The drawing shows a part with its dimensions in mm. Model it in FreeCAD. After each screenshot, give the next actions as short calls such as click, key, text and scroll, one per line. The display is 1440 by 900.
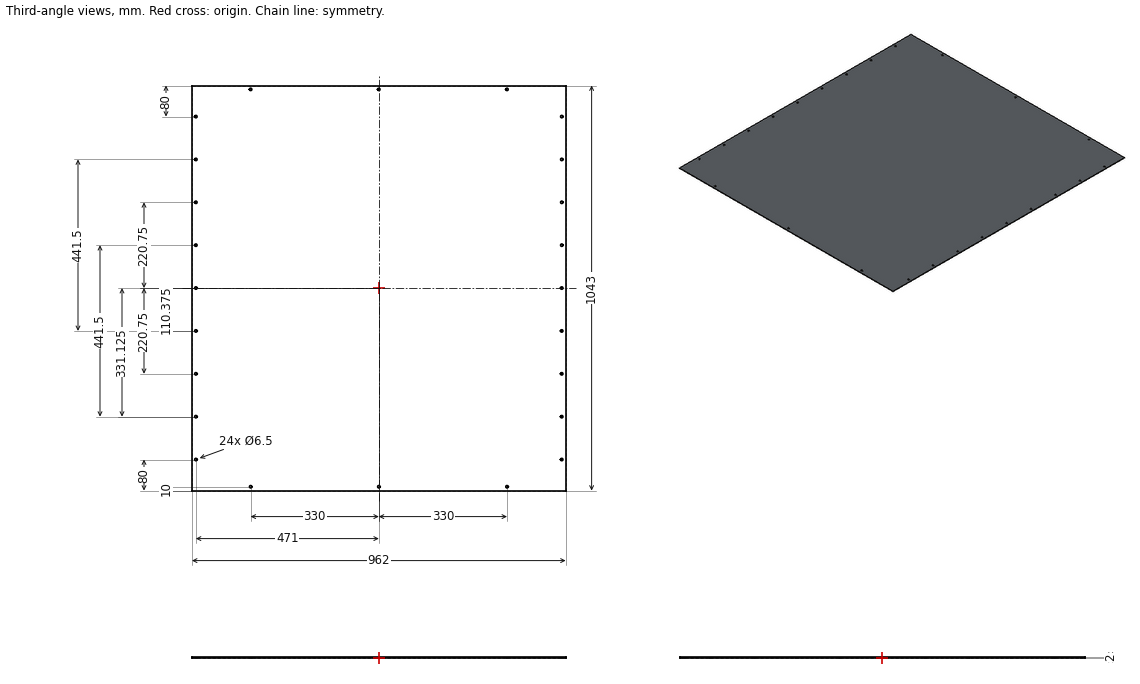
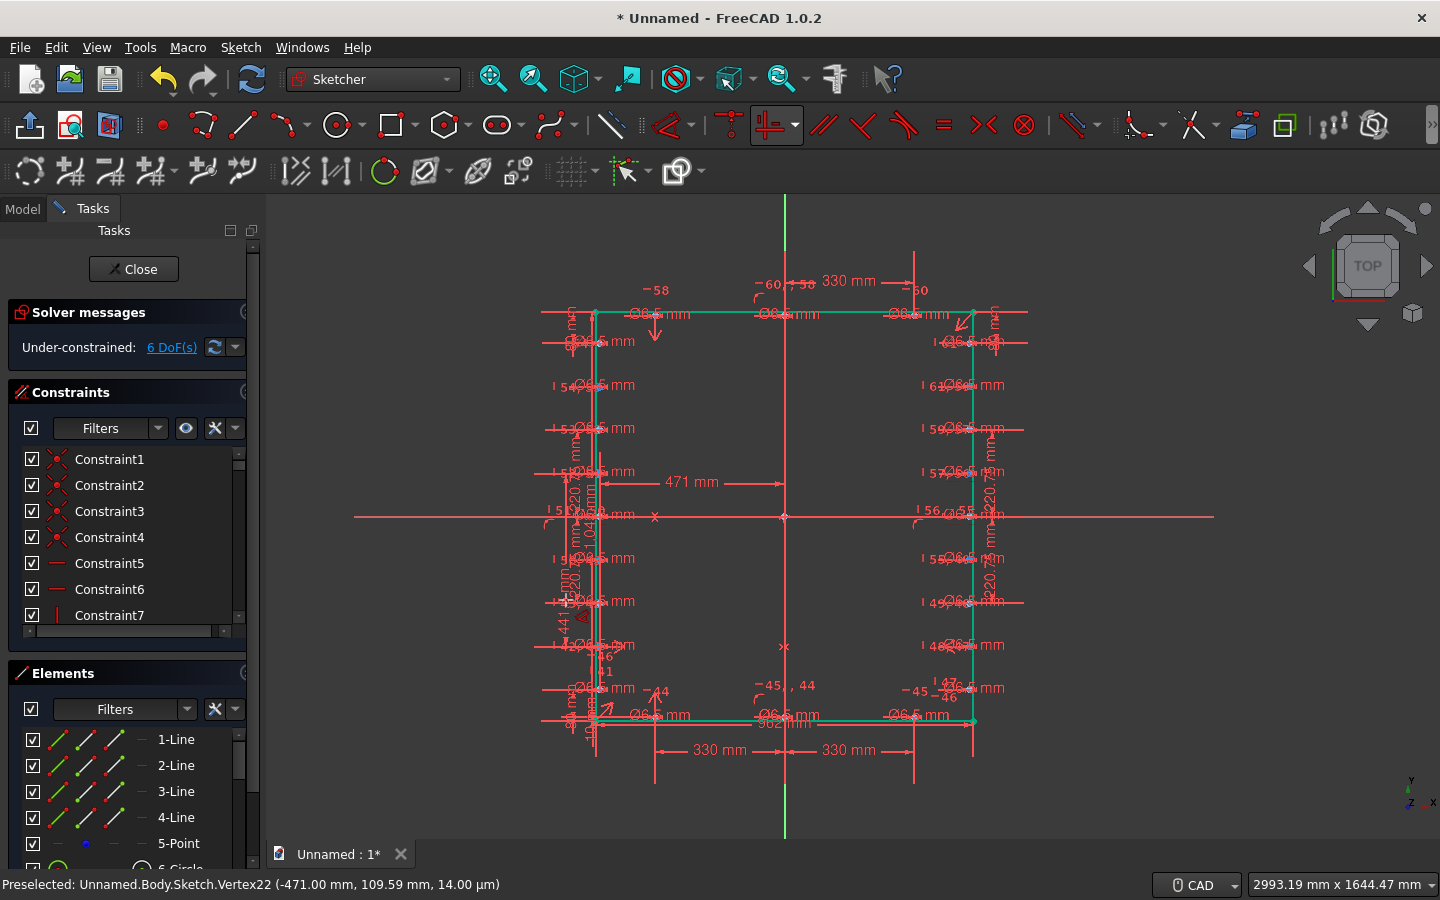
click(600, 560)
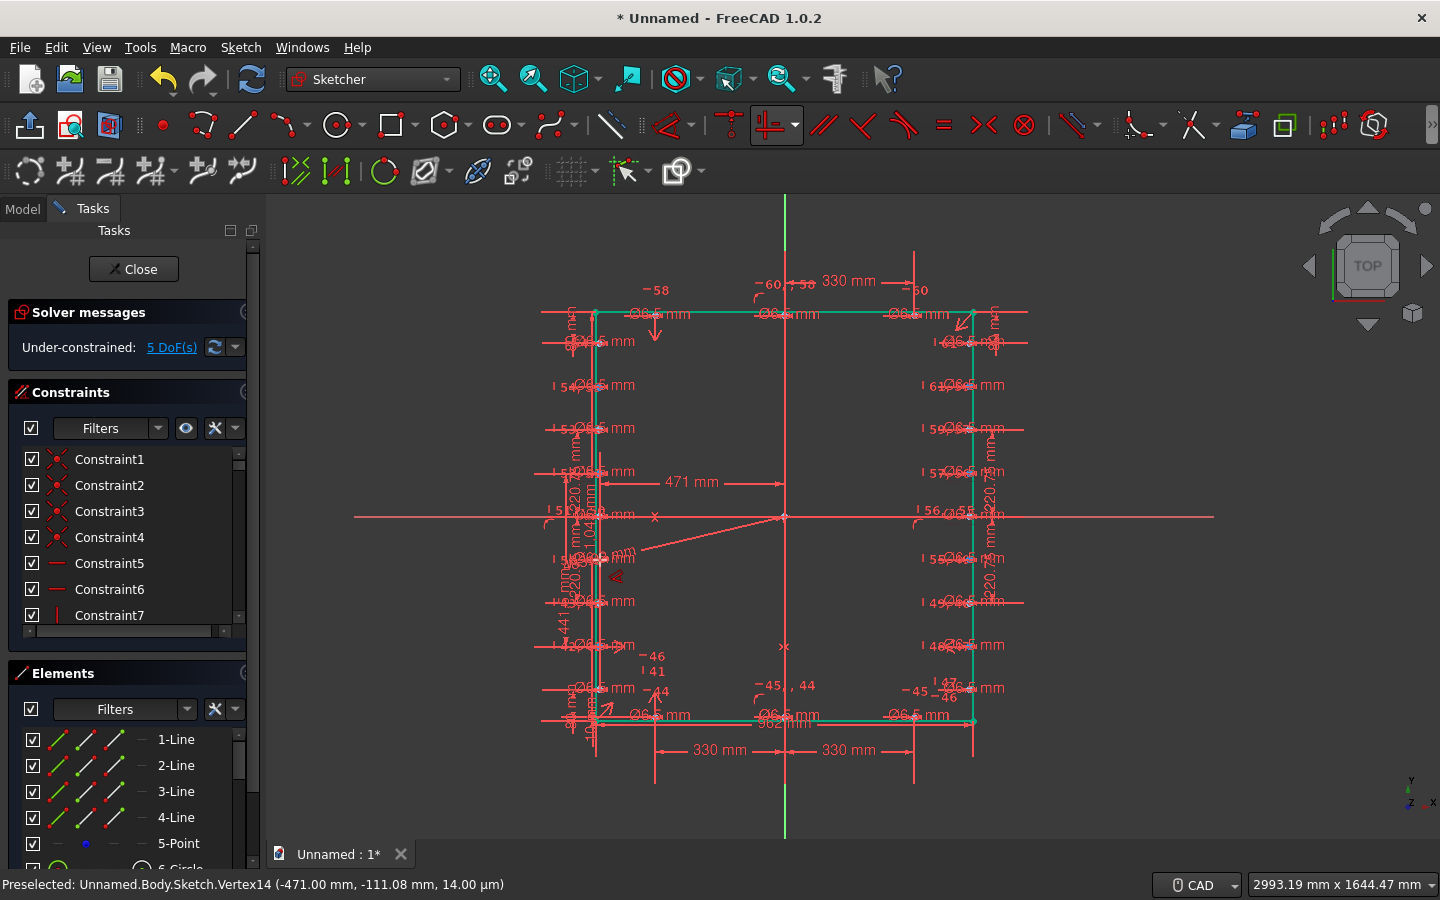
click(600, 387)
click(566, 434)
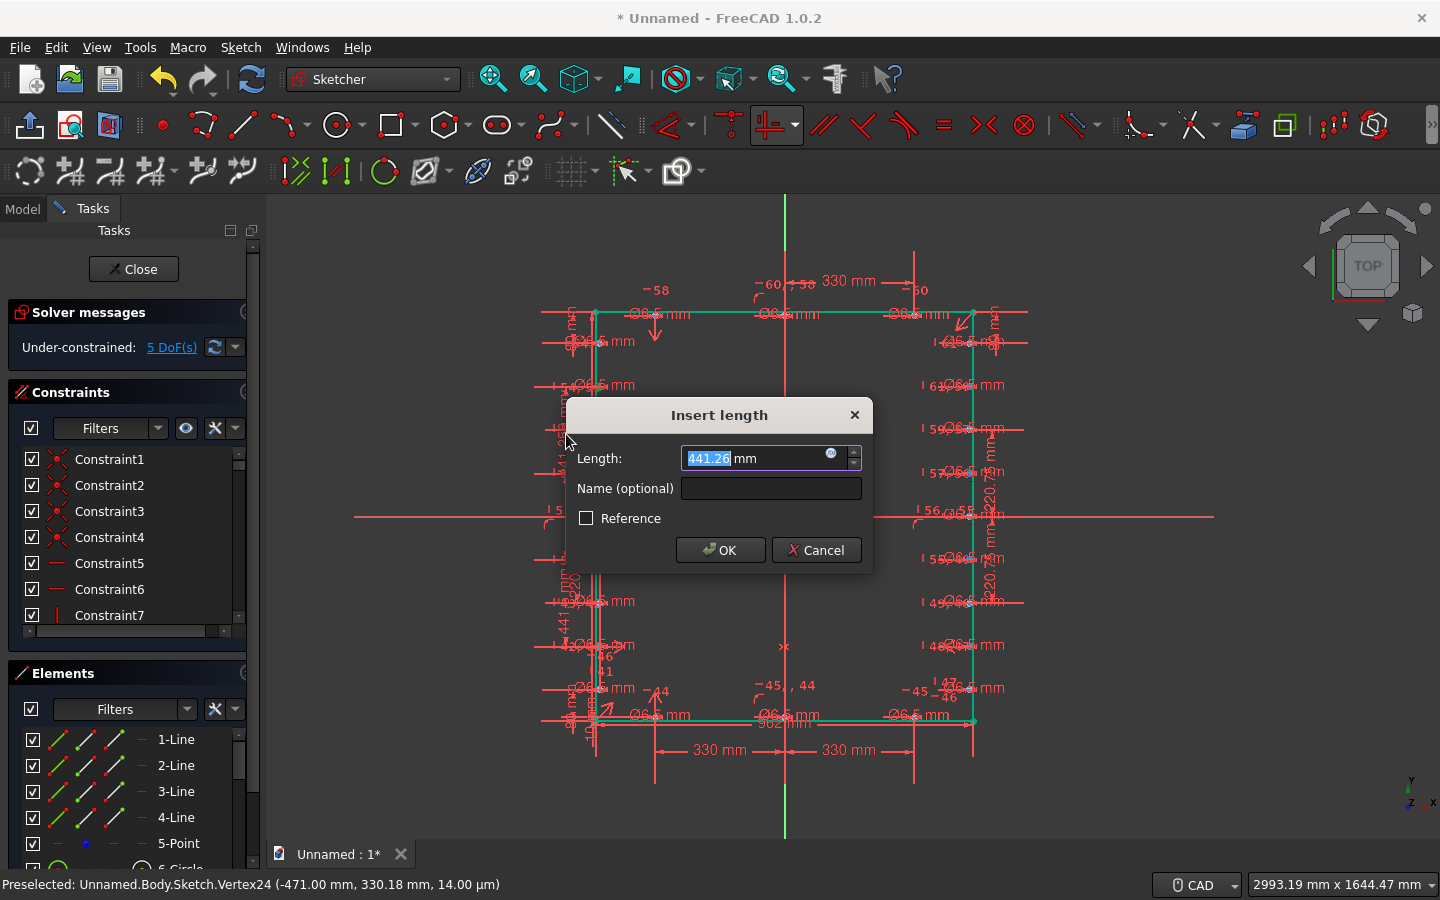
text(441.5)
key(Return)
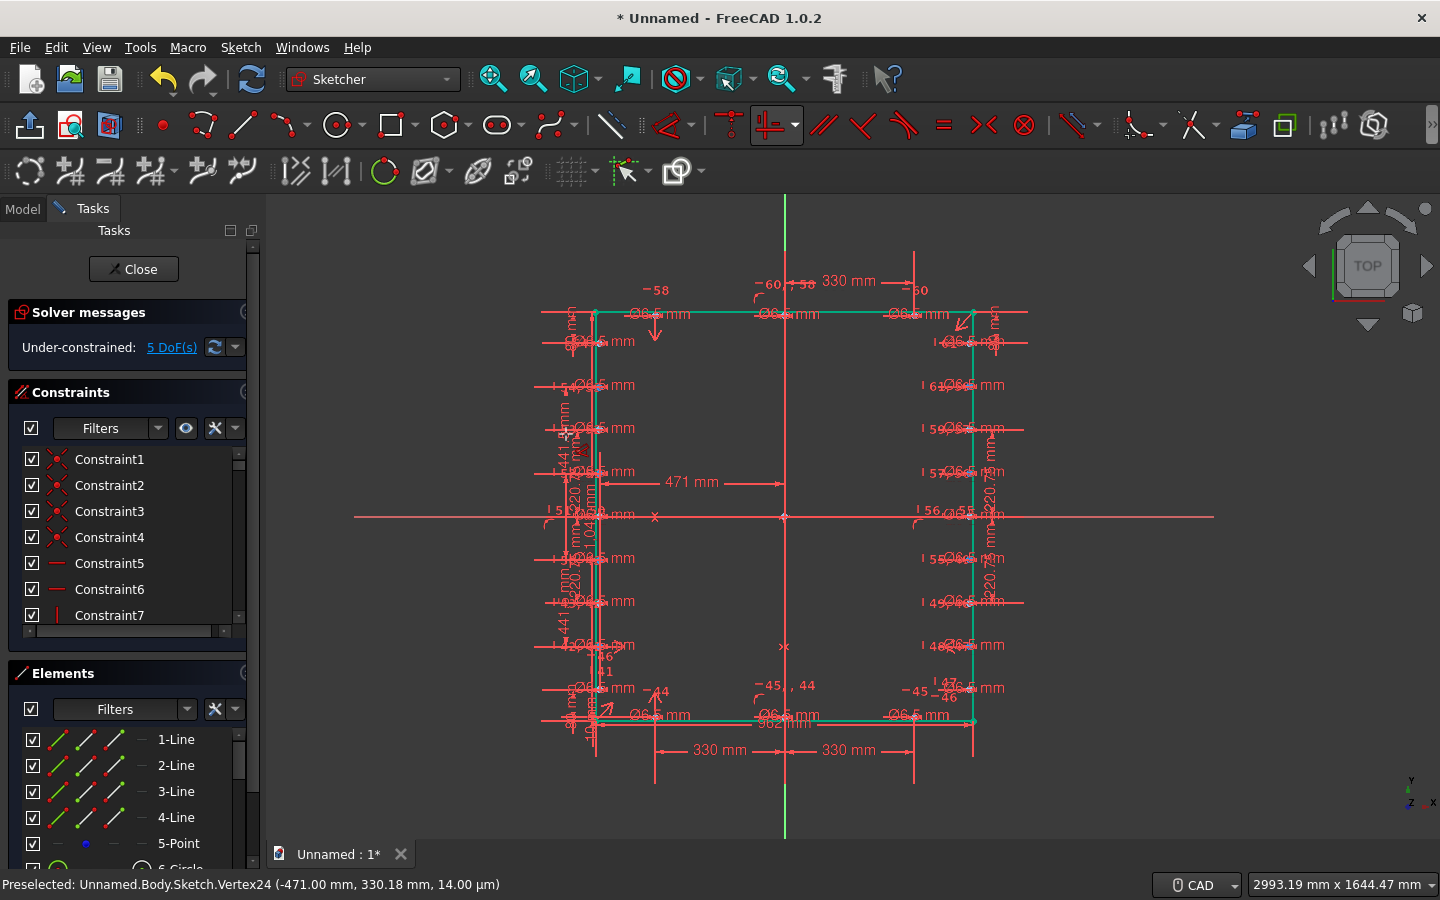
click(969, 647)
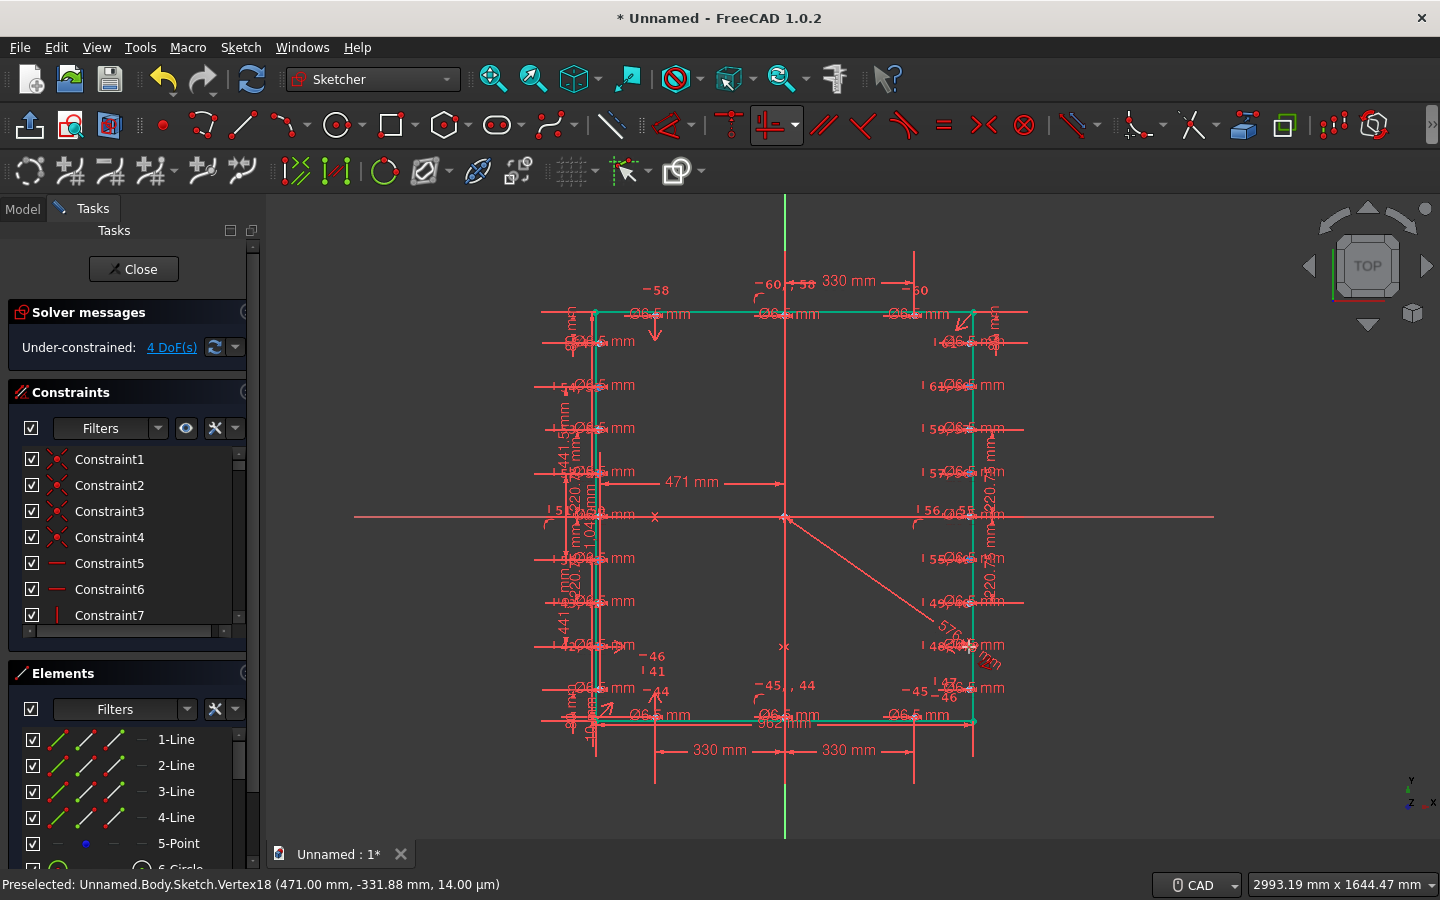
click(969, 474)
click(1003, 600)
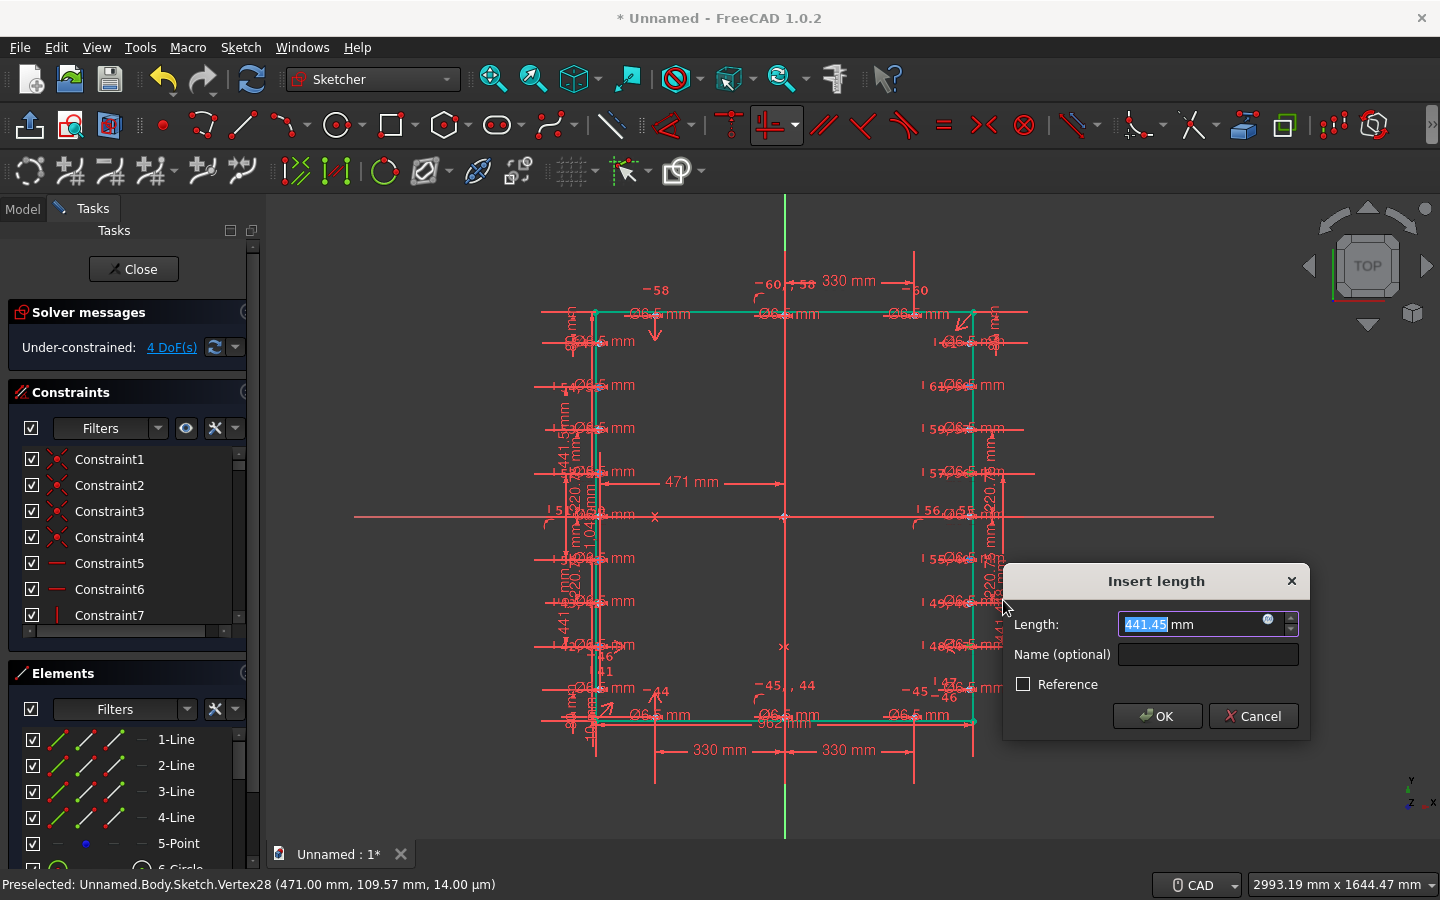
text(441.5)
key(Return)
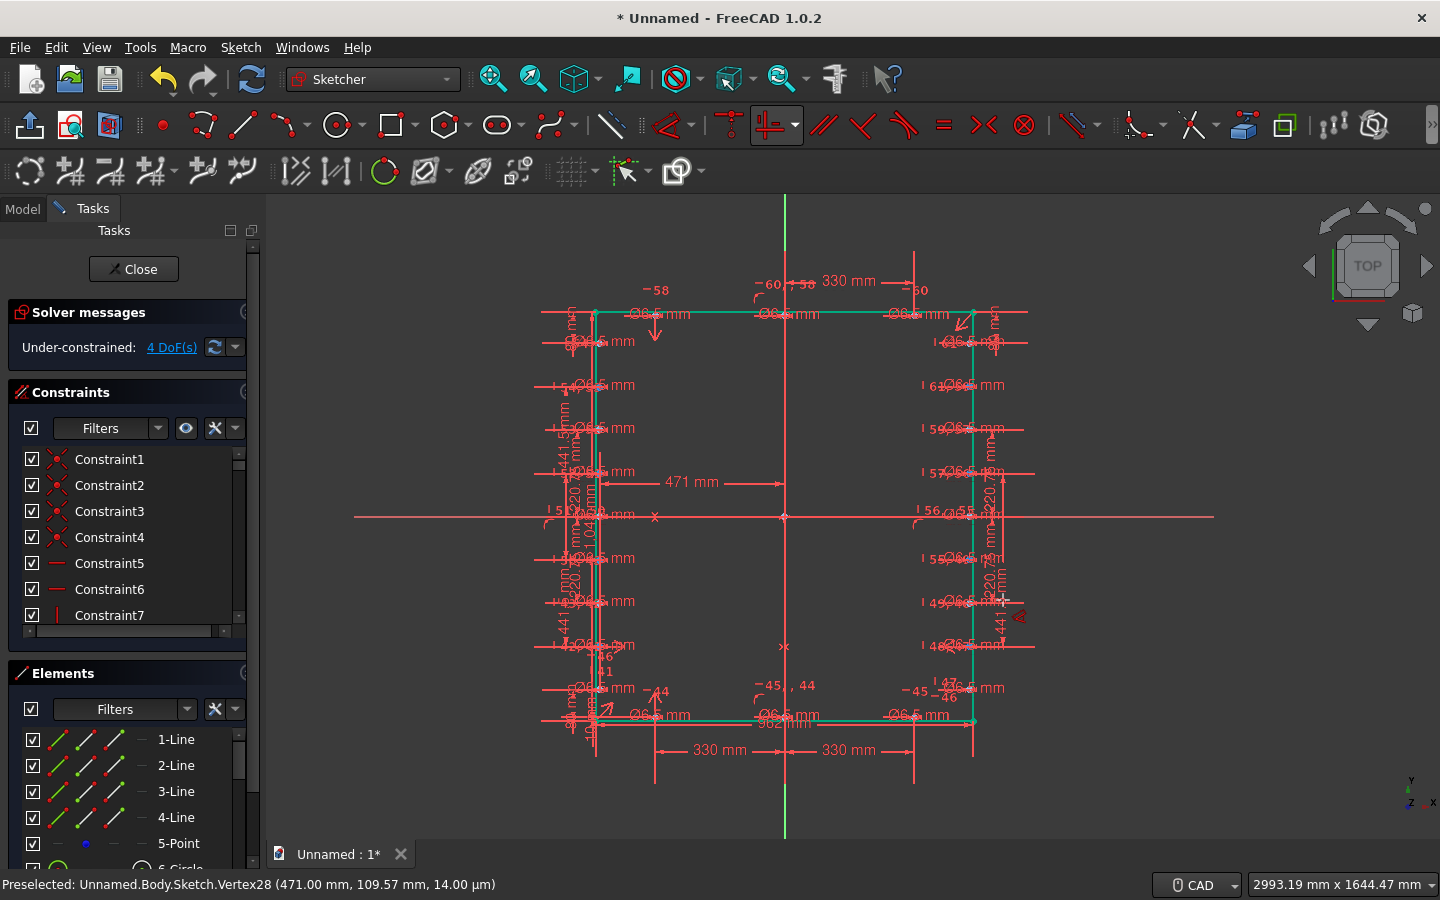
click(969, 560)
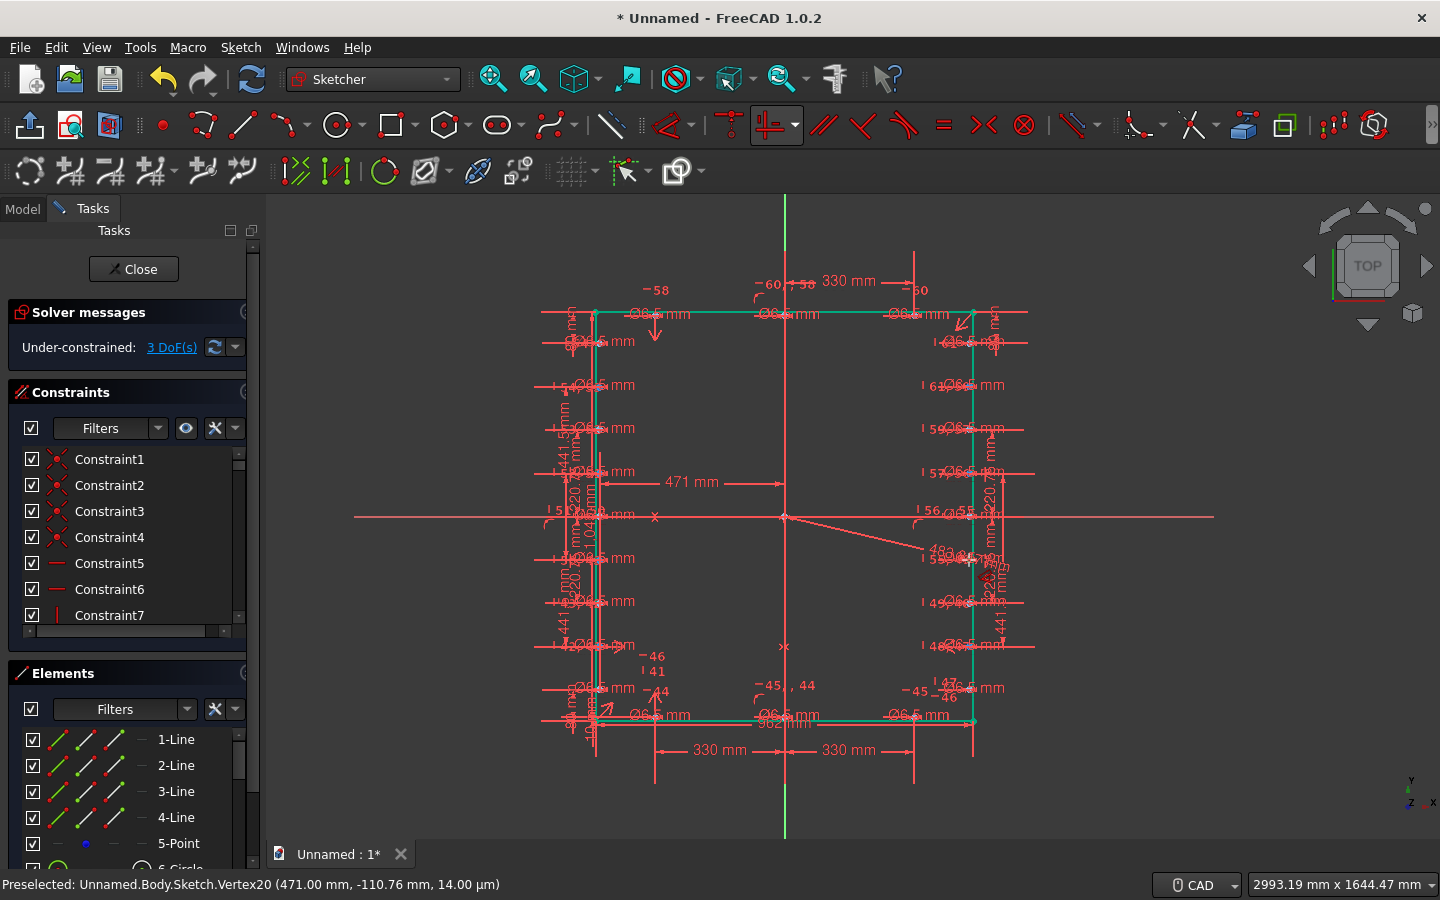
click(969, 387)
click(1003, 434)